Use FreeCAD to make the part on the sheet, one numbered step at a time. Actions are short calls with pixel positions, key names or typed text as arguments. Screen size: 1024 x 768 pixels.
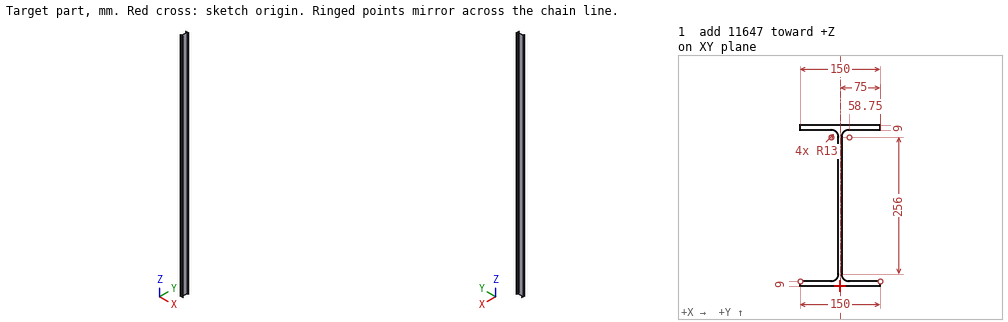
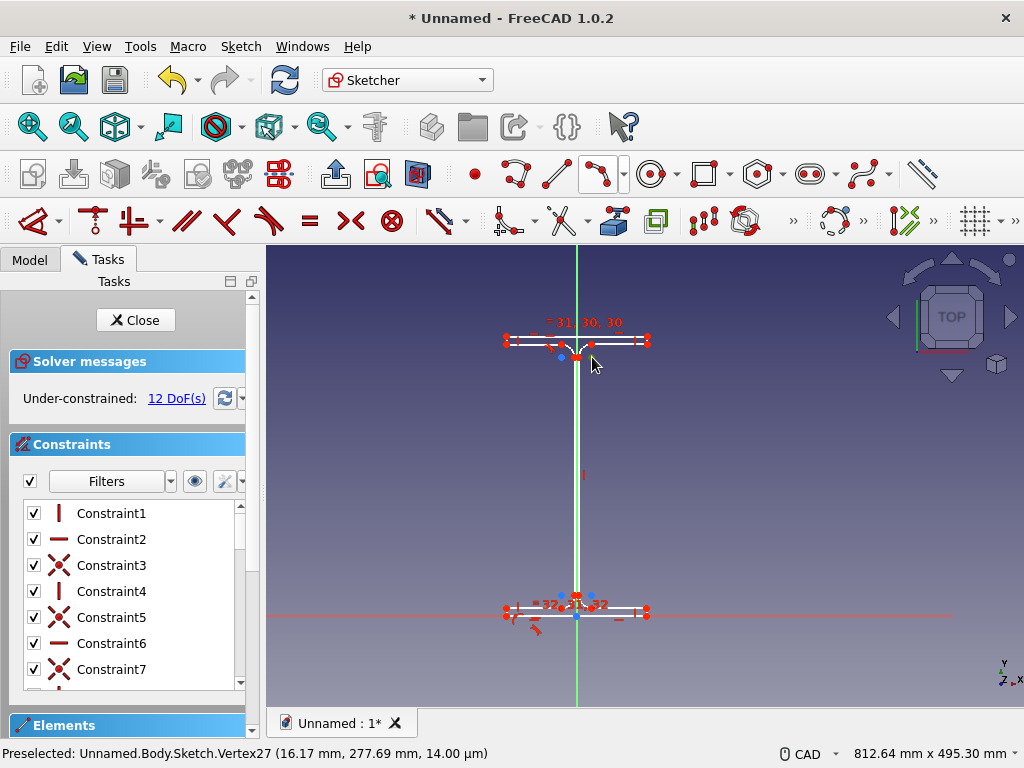
click(562, 358)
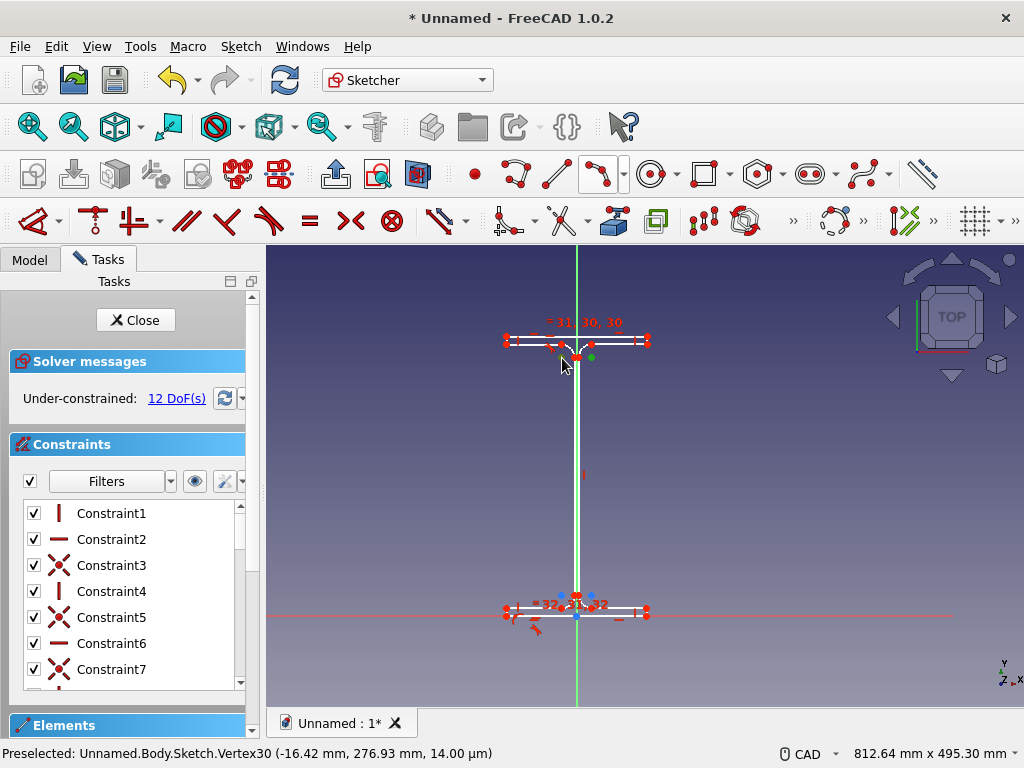
click(577, 650)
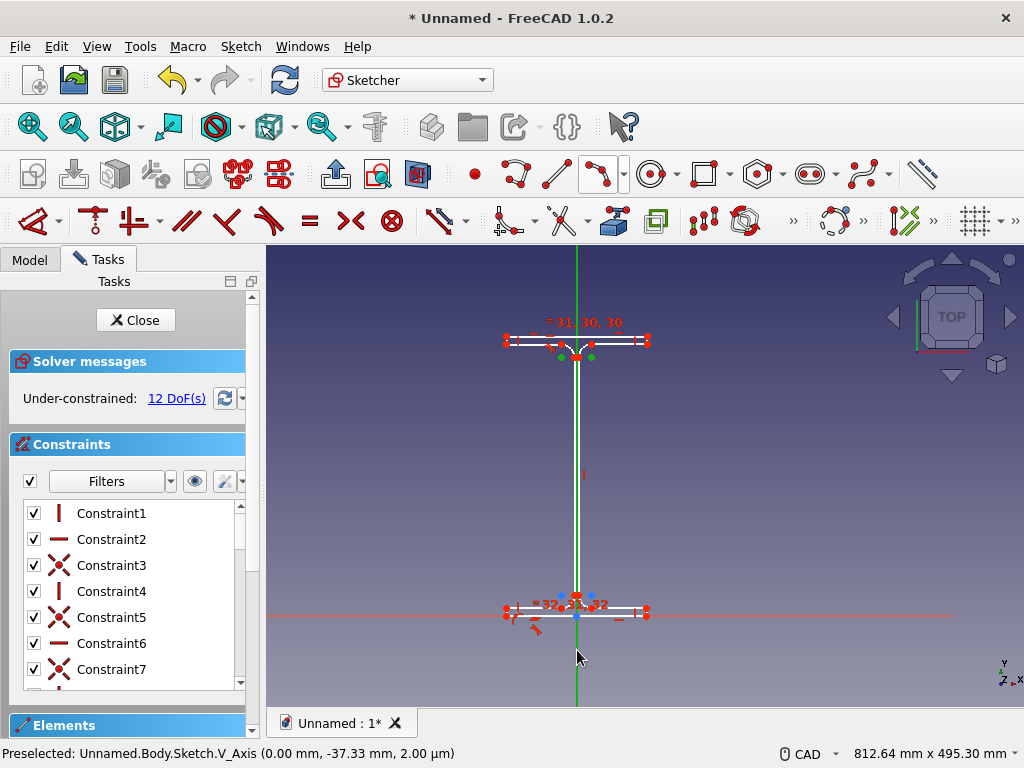
click(351, 222)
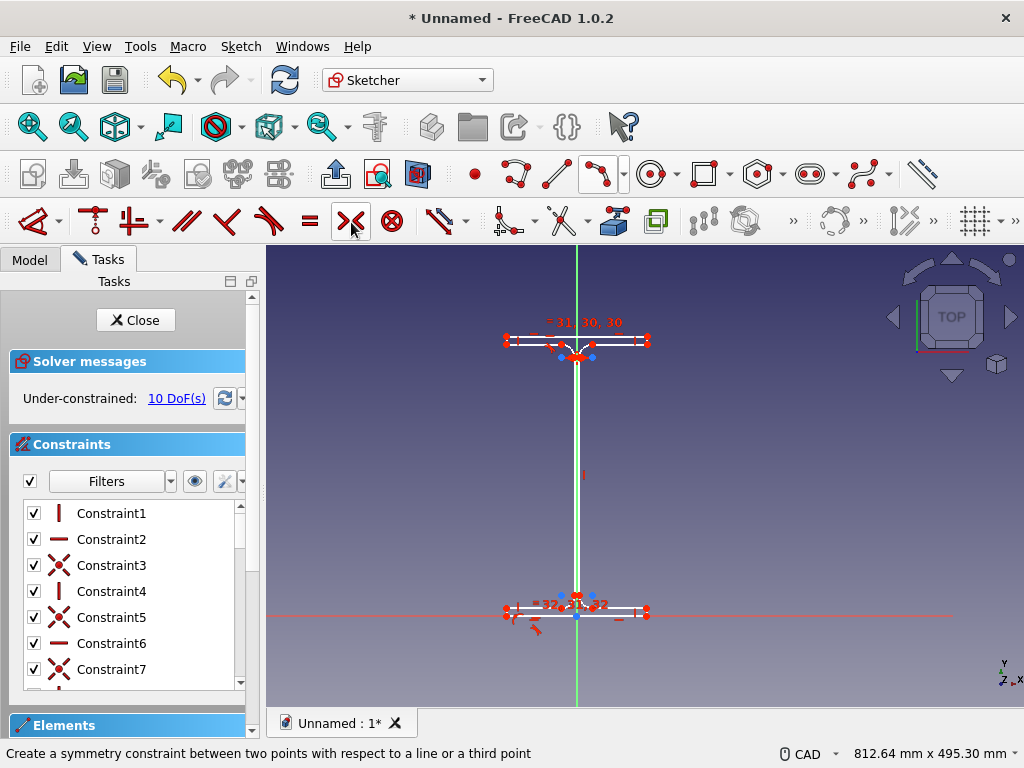
scroll(507, 608, up, 3)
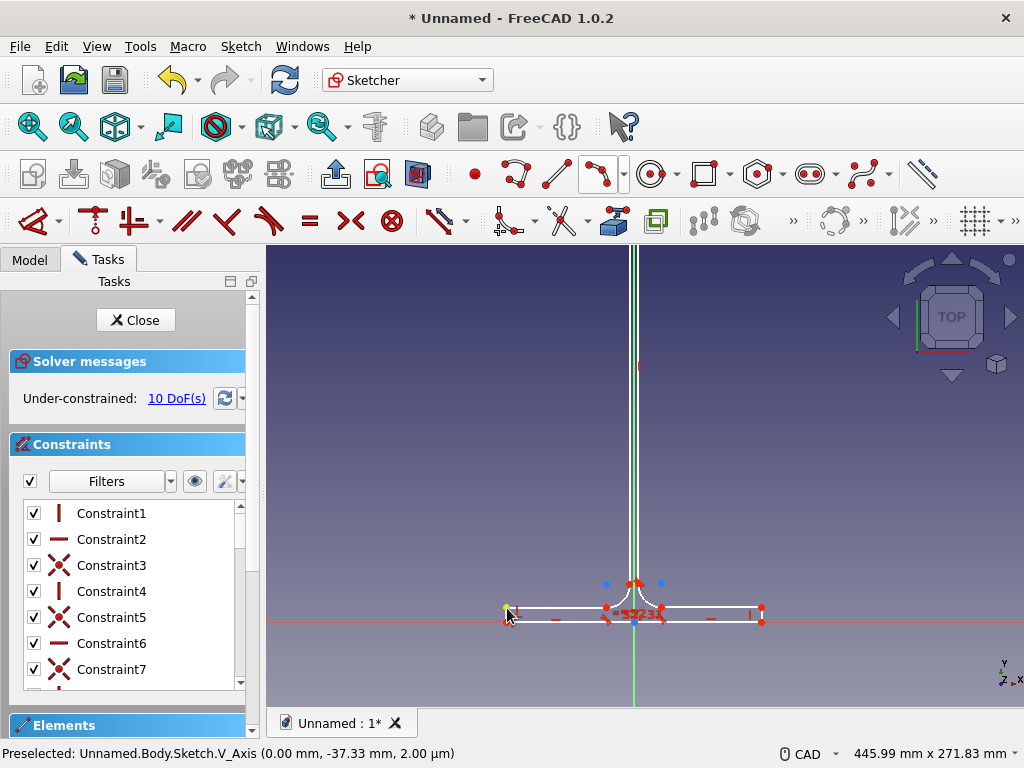
click(506, 608)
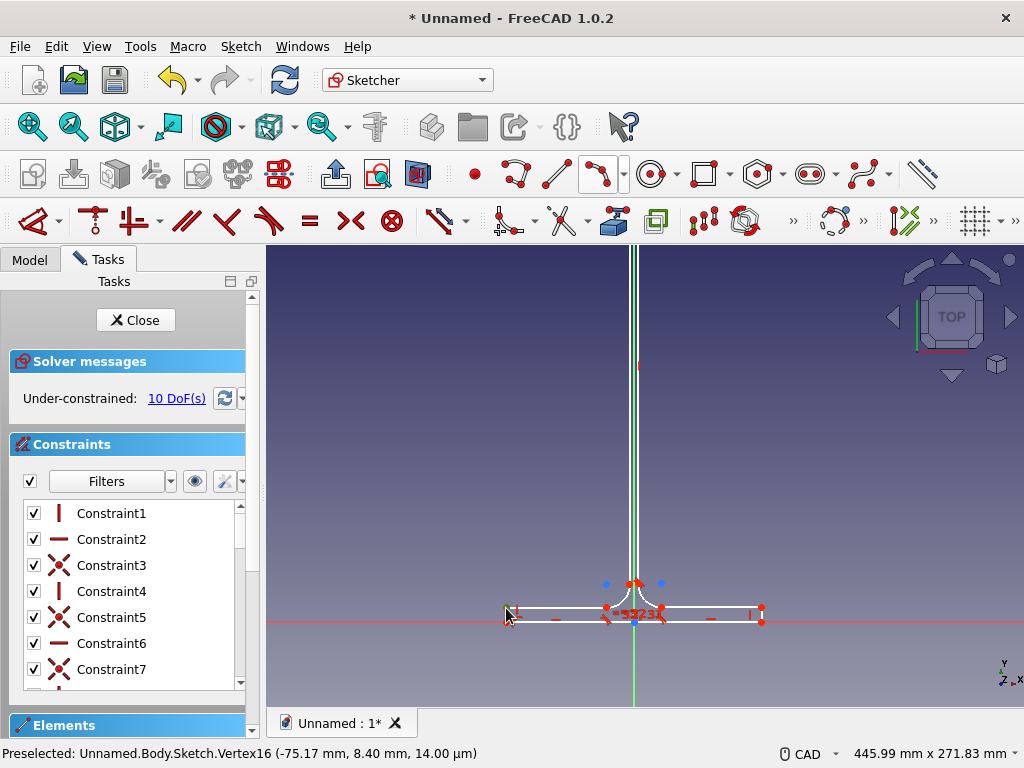
click(762, 607)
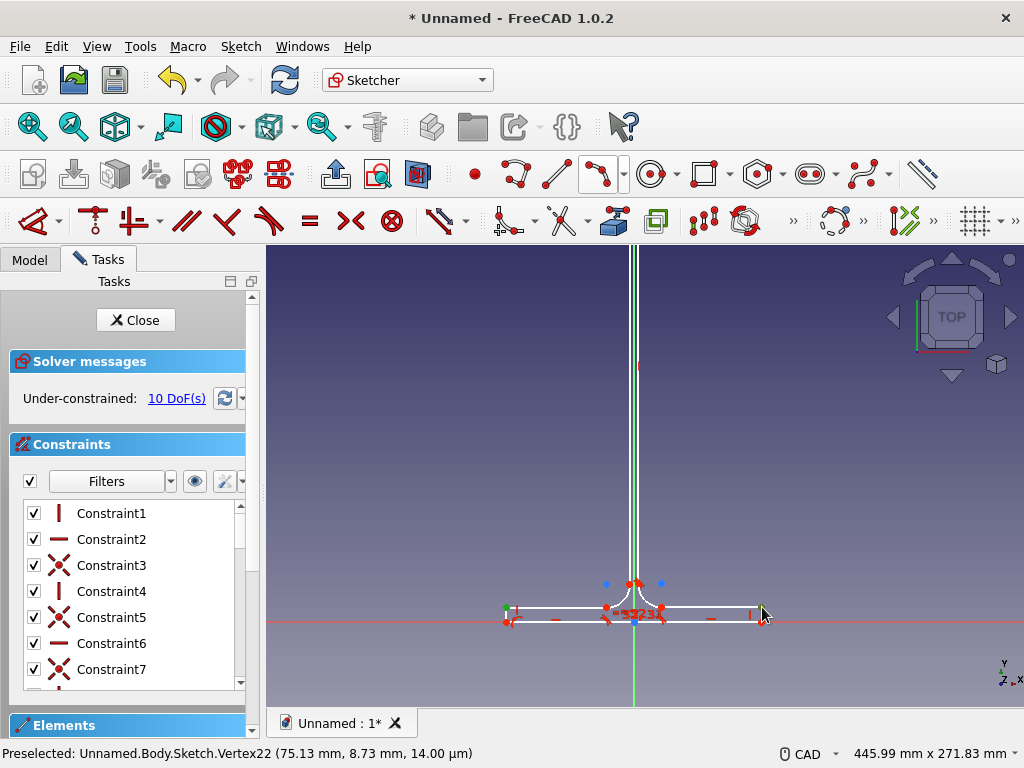
click(634, 650)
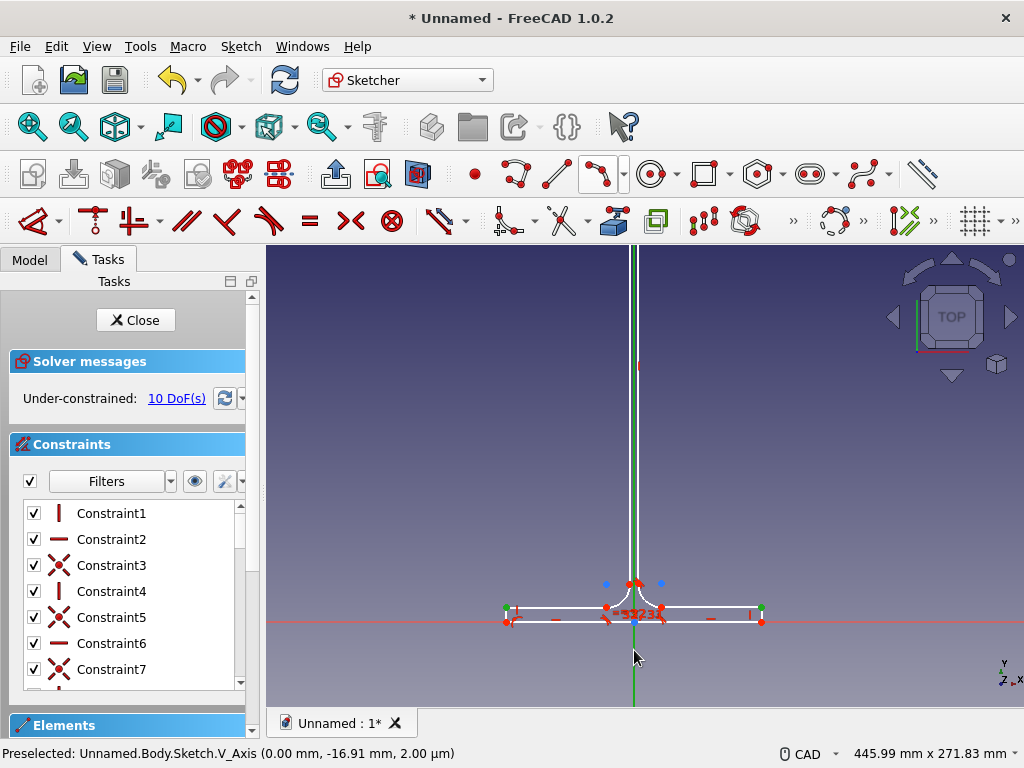
key(s)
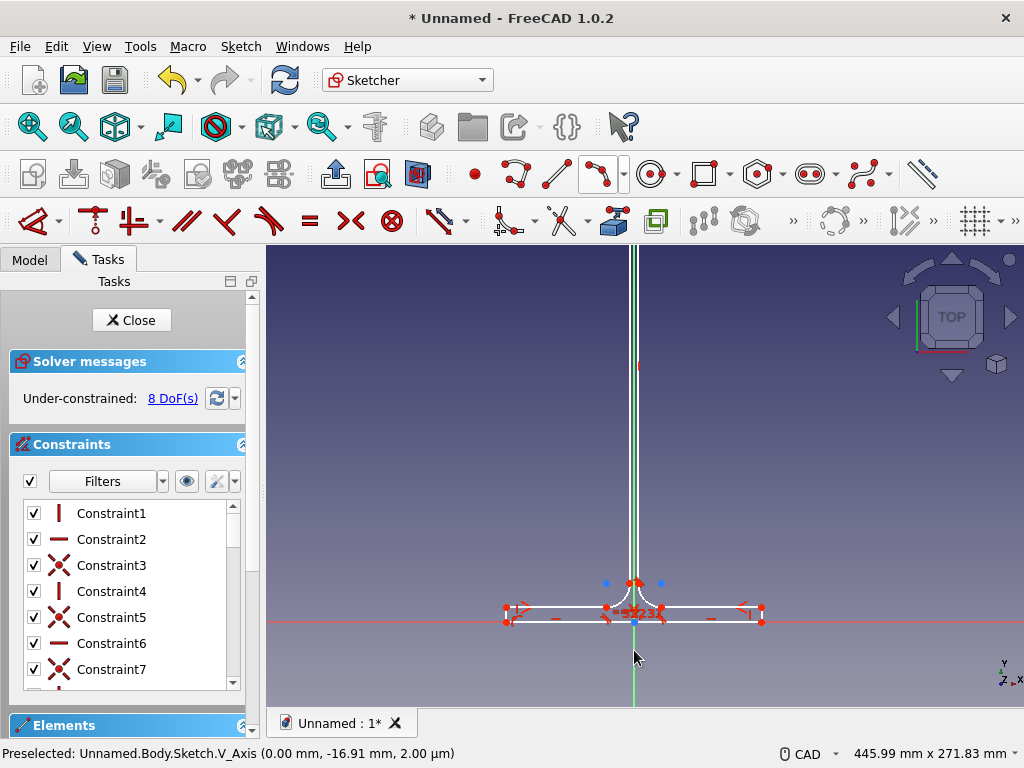
click(32, 222)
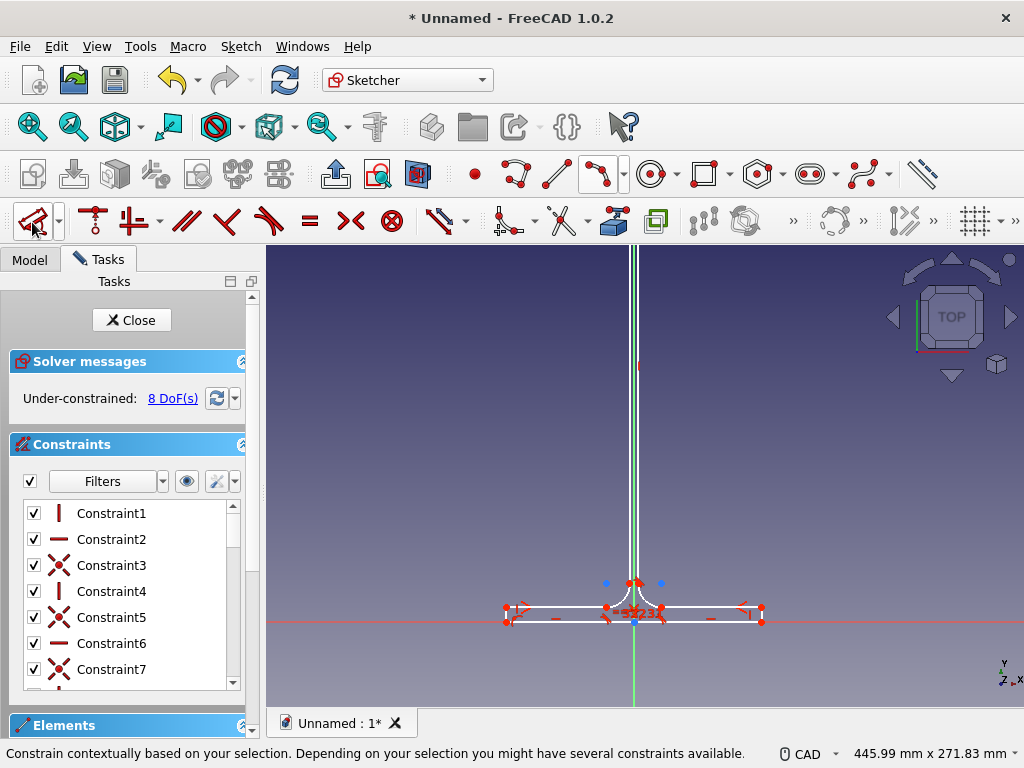
scroll(506, 608, down, 3)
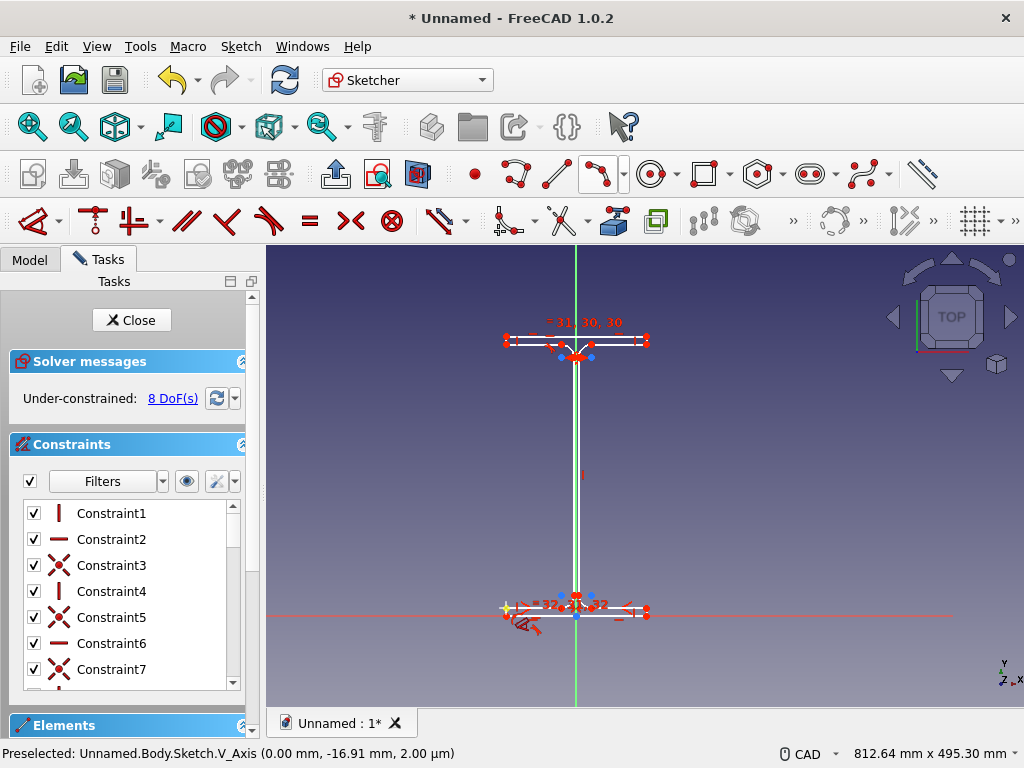
scroll(586, 346, up, 6)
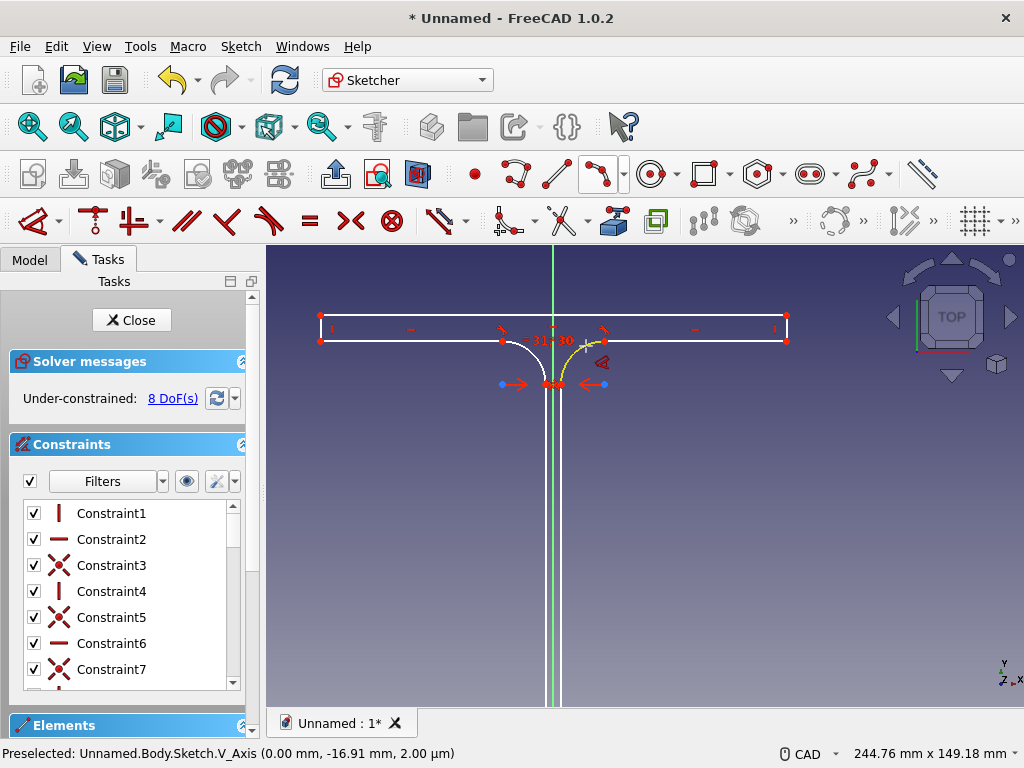
click(585, 346)
click(530, 376)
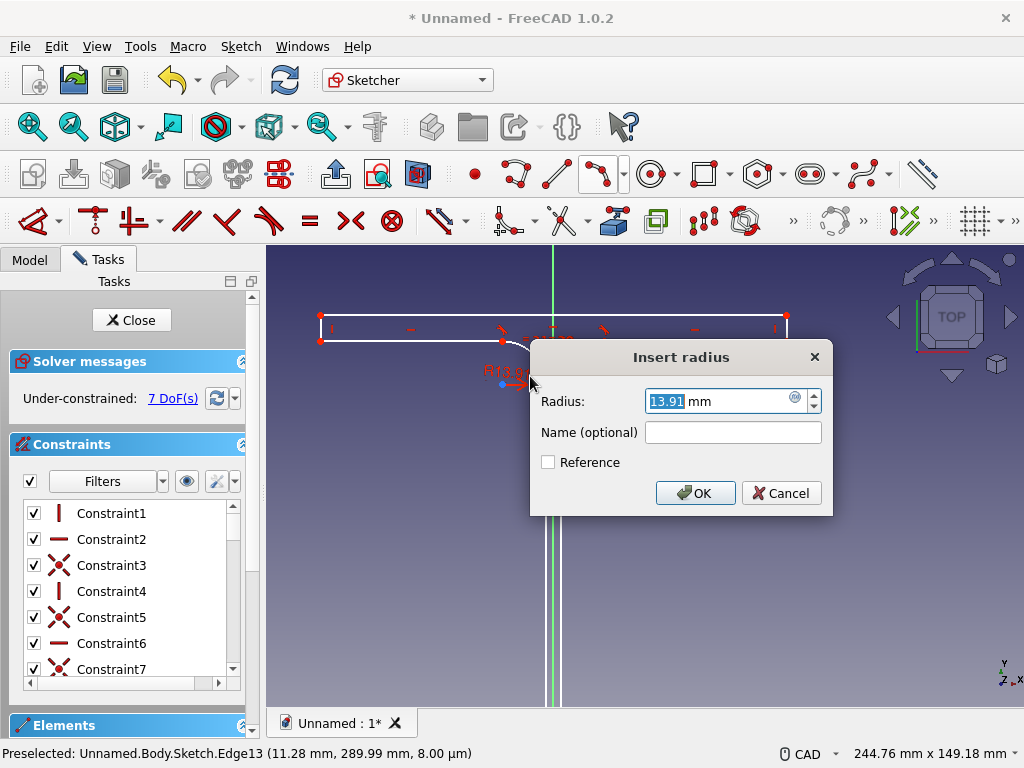
text(13)
key(Return)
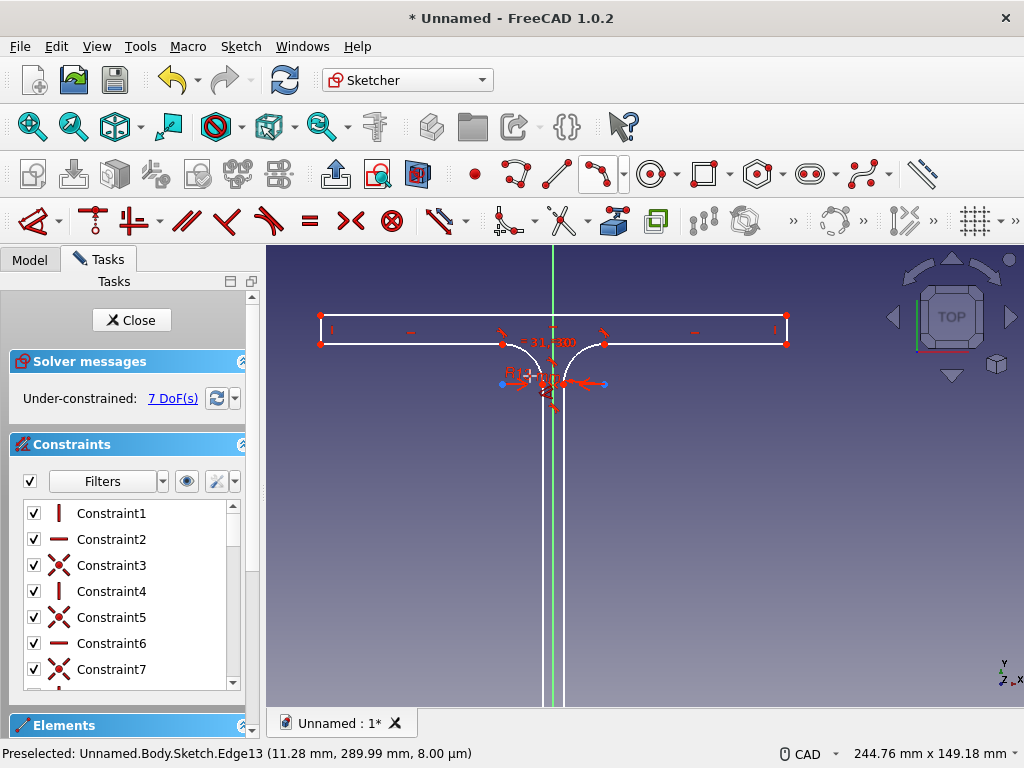
scroll(787, 333, up, 2)